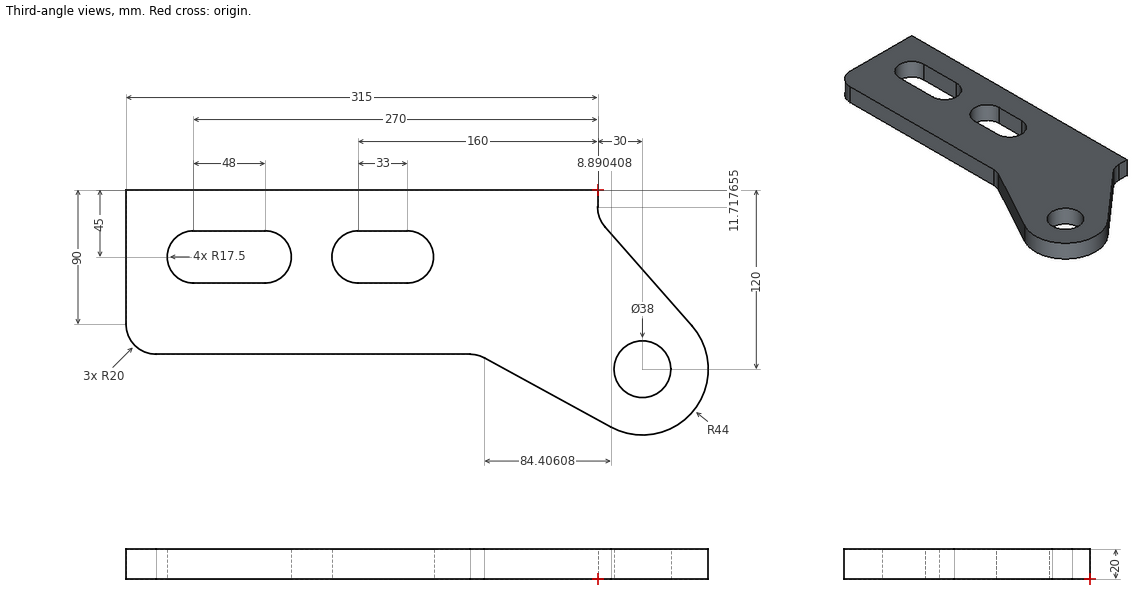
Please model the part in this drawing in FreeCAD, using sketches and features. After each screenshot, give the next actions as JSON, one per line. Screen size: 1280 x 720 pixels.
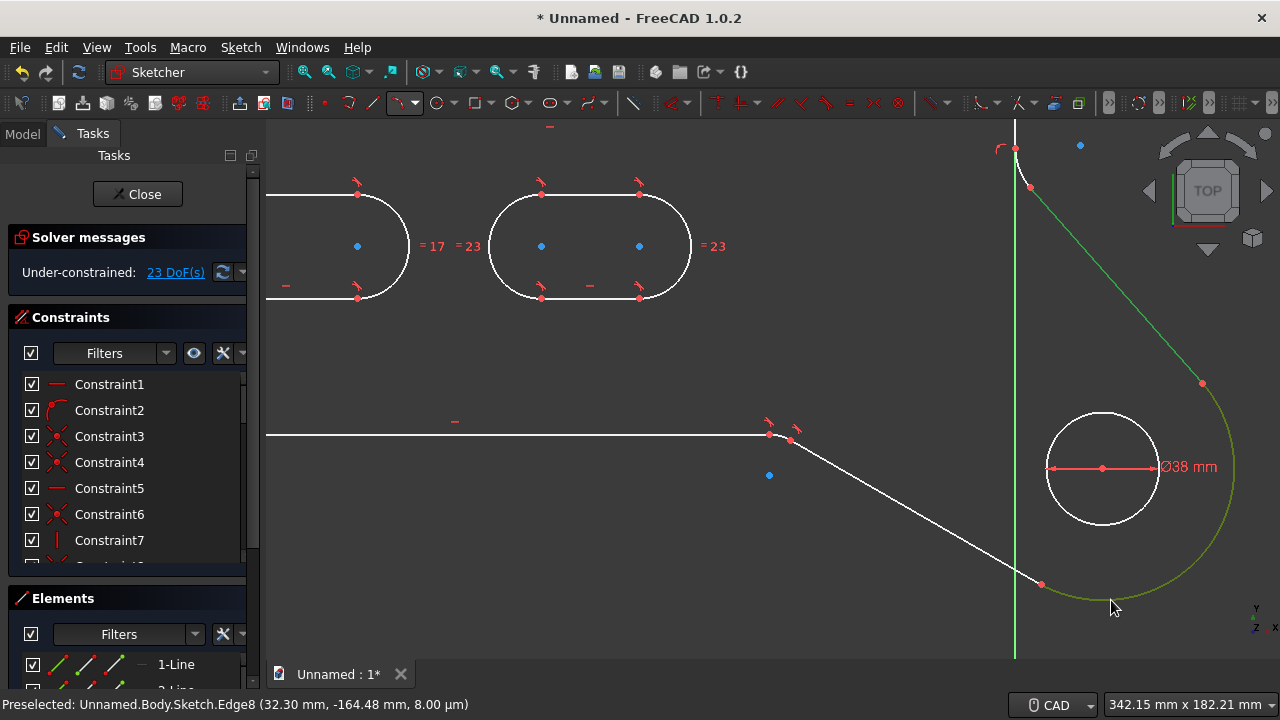
{"action": "left_click", "coordinate": [826, 104]}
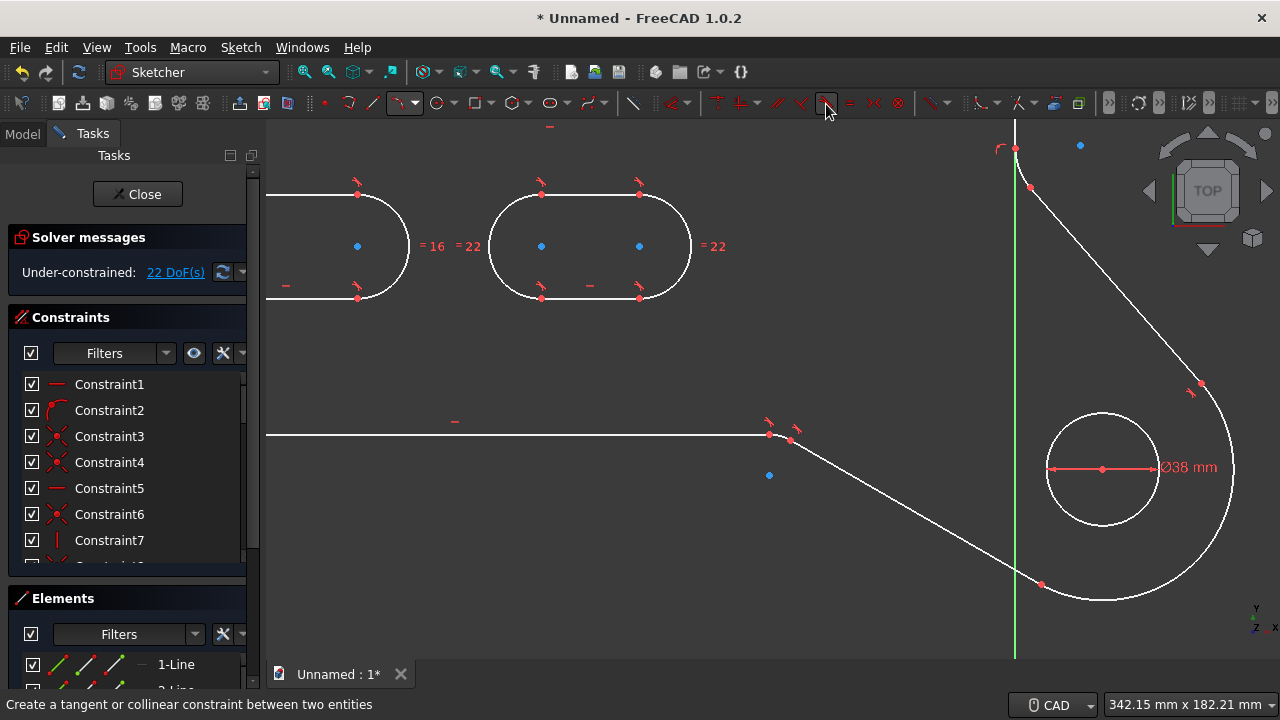
{"action": "left_click", "coordinate": [1081, 246]}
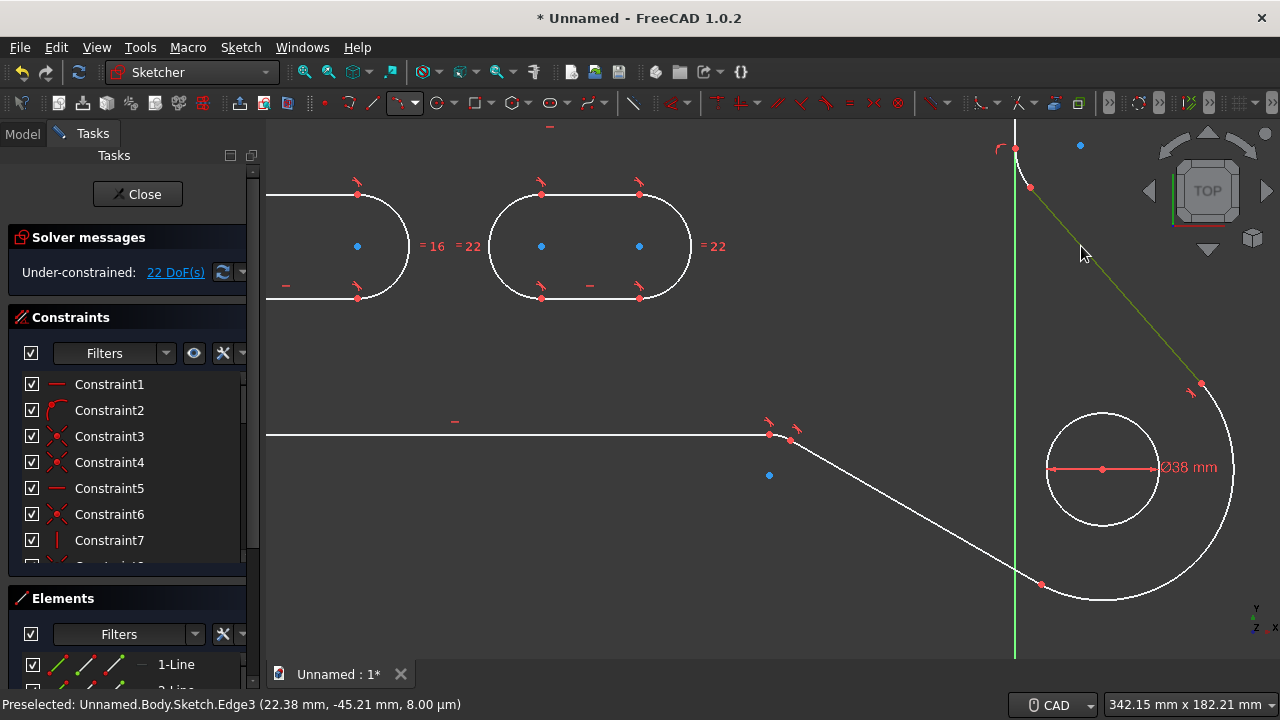
{"action": "left_click", "coordinate": [1017, 161]}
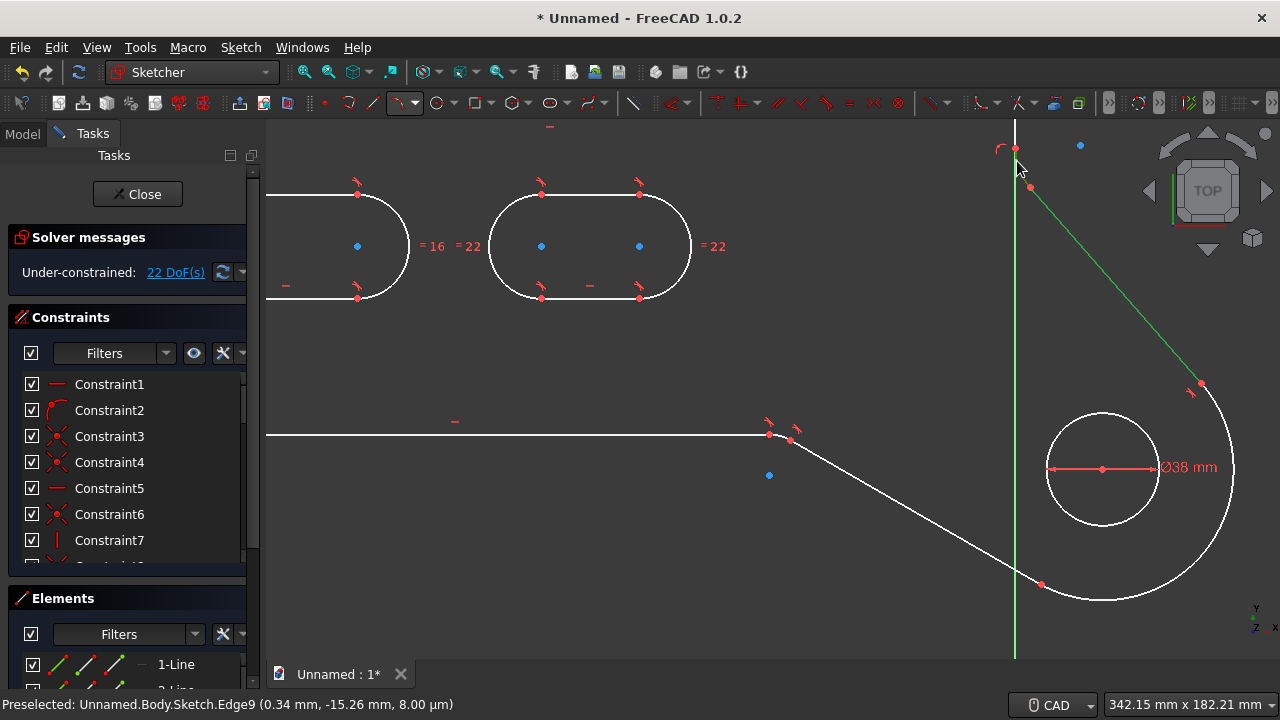
{"action": "key", "text": "t"}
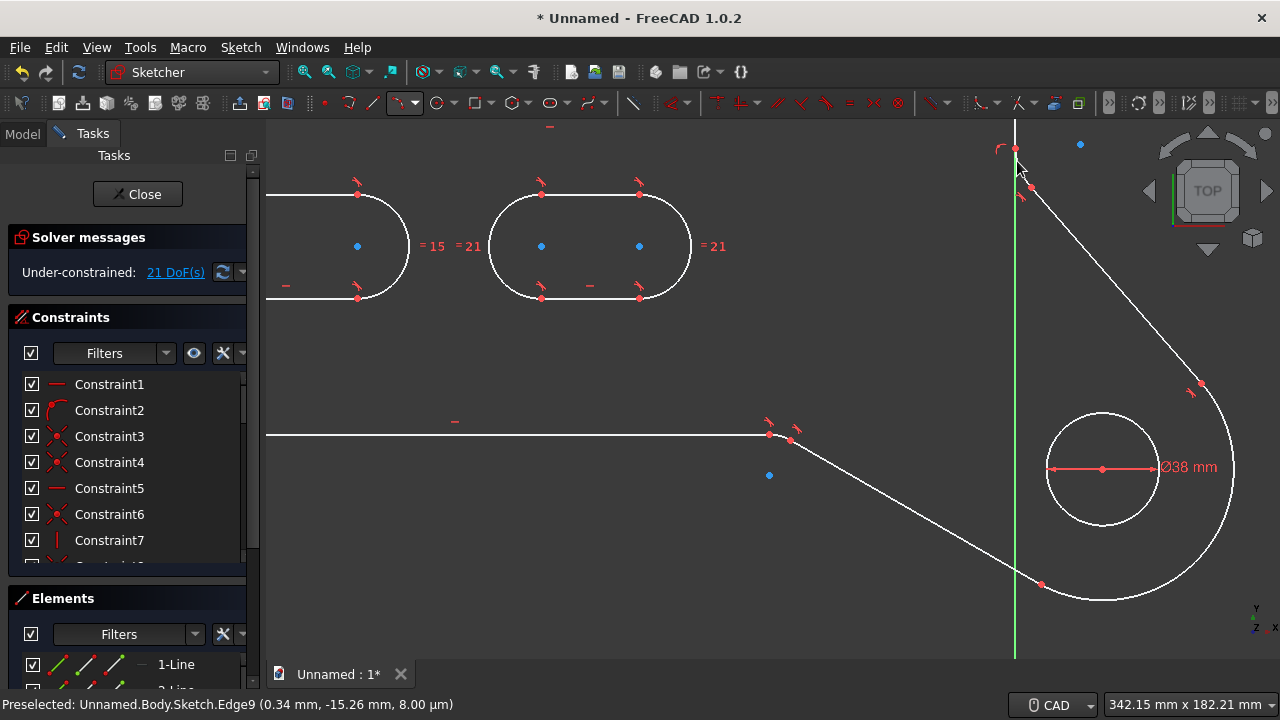
{"action": "scroll", "coordinate": [778, 439], "scroll_direction": "down", "scroll_amount": 3}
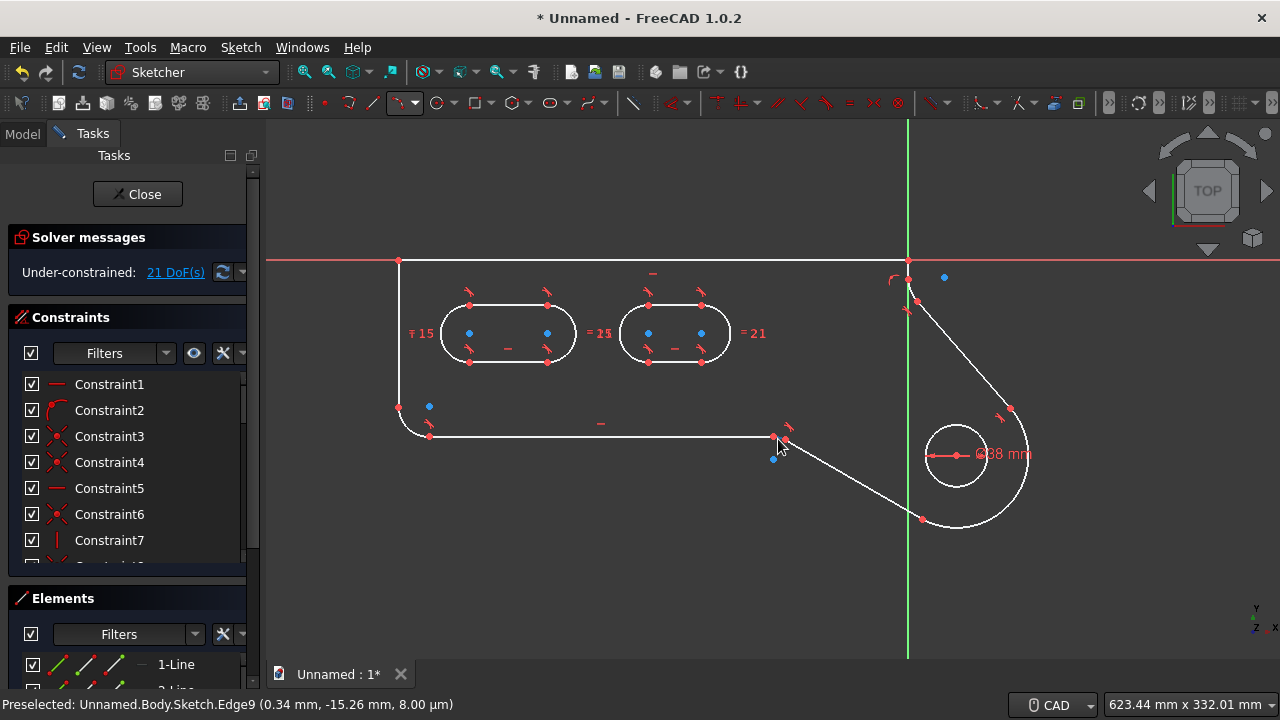
{"action": "scroll", "coordinate": [908, 274], "scroll_direction": "up", "scroll_amount": 5}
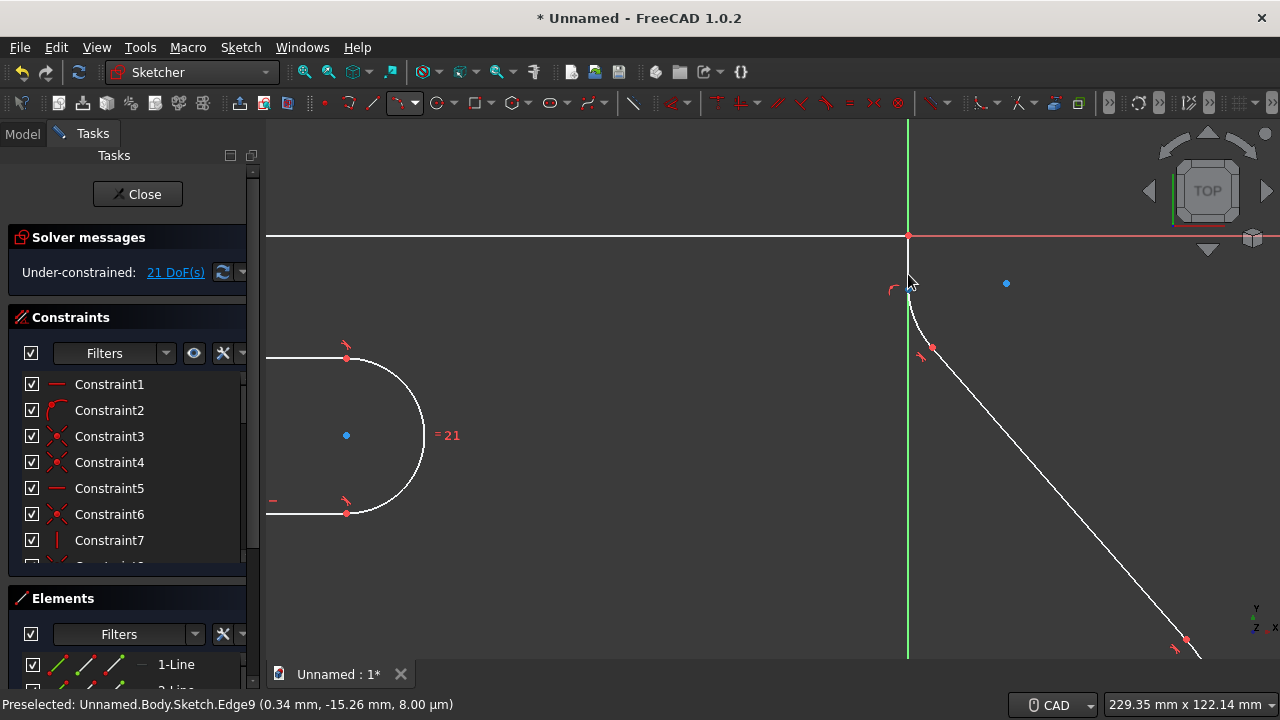
{"action": "left_click", "coordinate": [908, 273]}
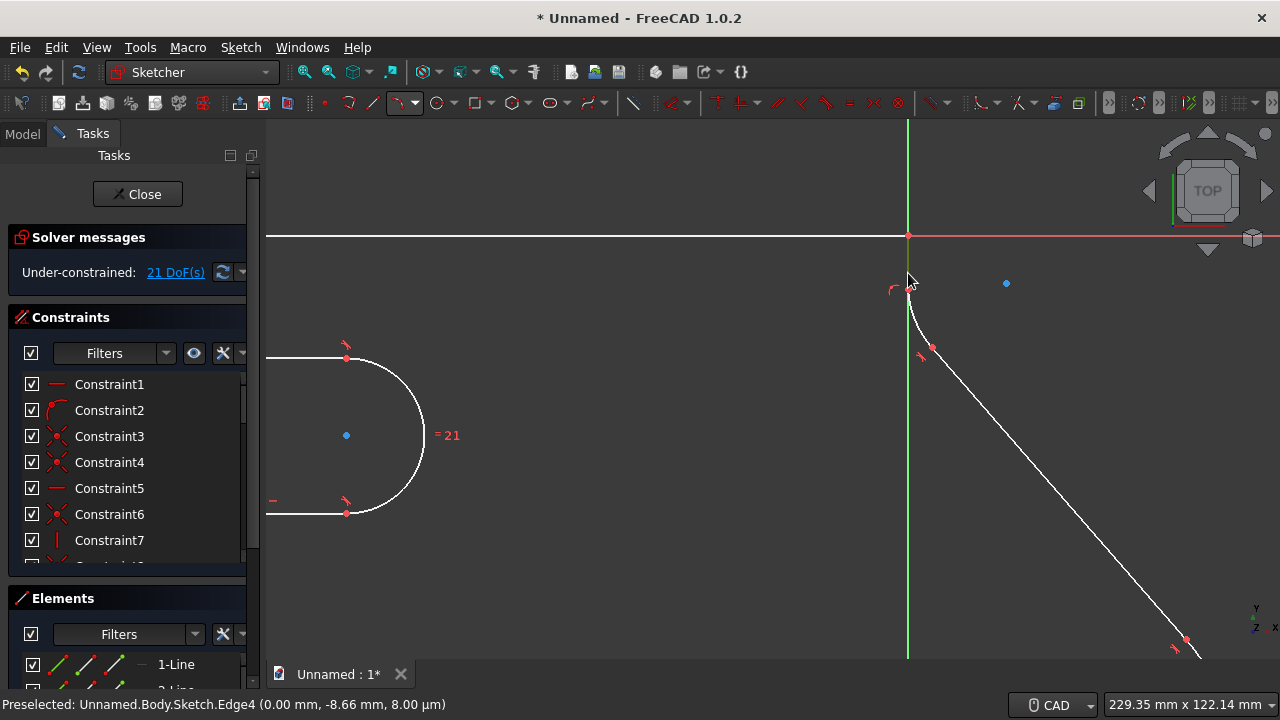
{"action": "left_click", "coordinate": [911, 308]}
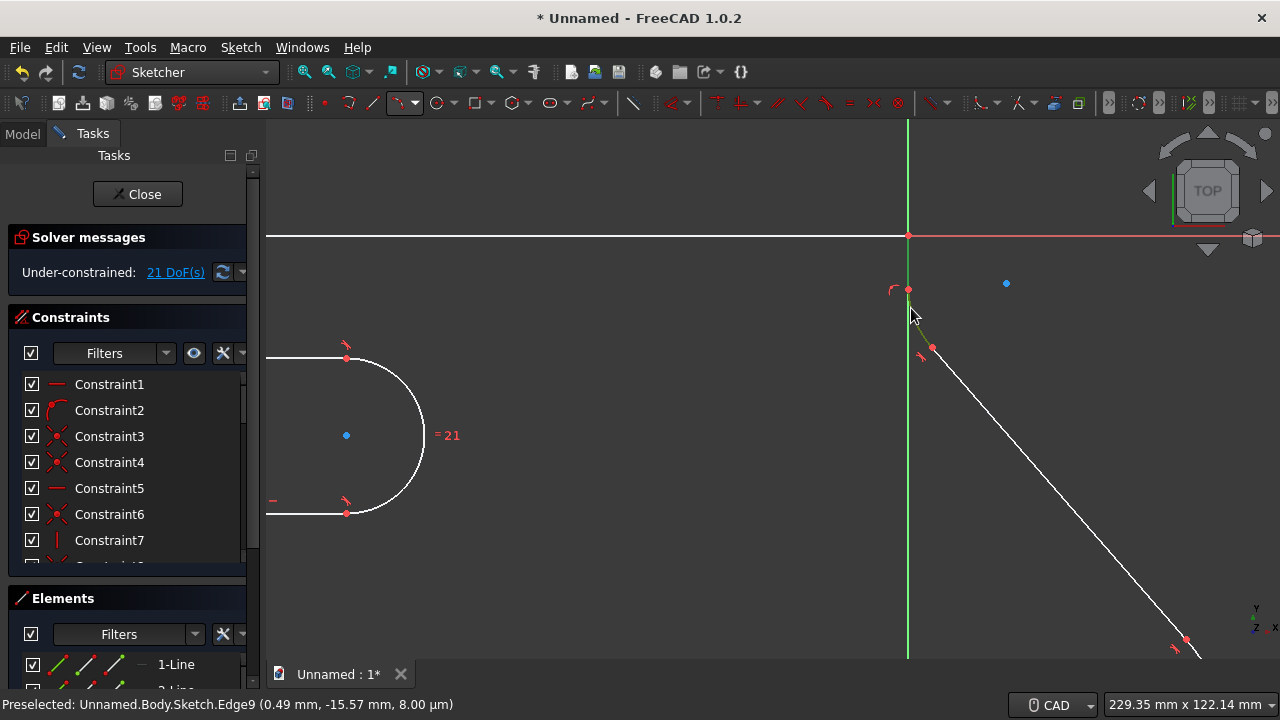
{"action": "key", "text": "t"}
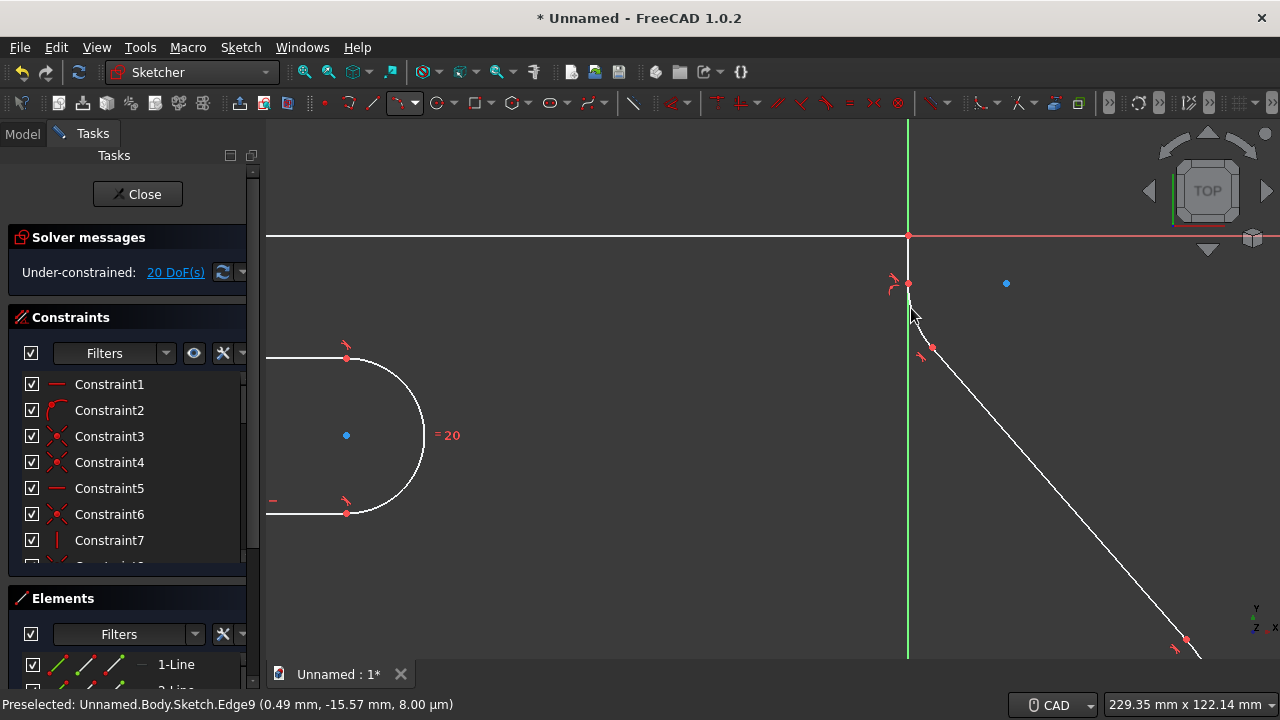
{"action": "scroll", "coordinate": [908, 274], "scroll_direction": "down", "scroll_amount": 5}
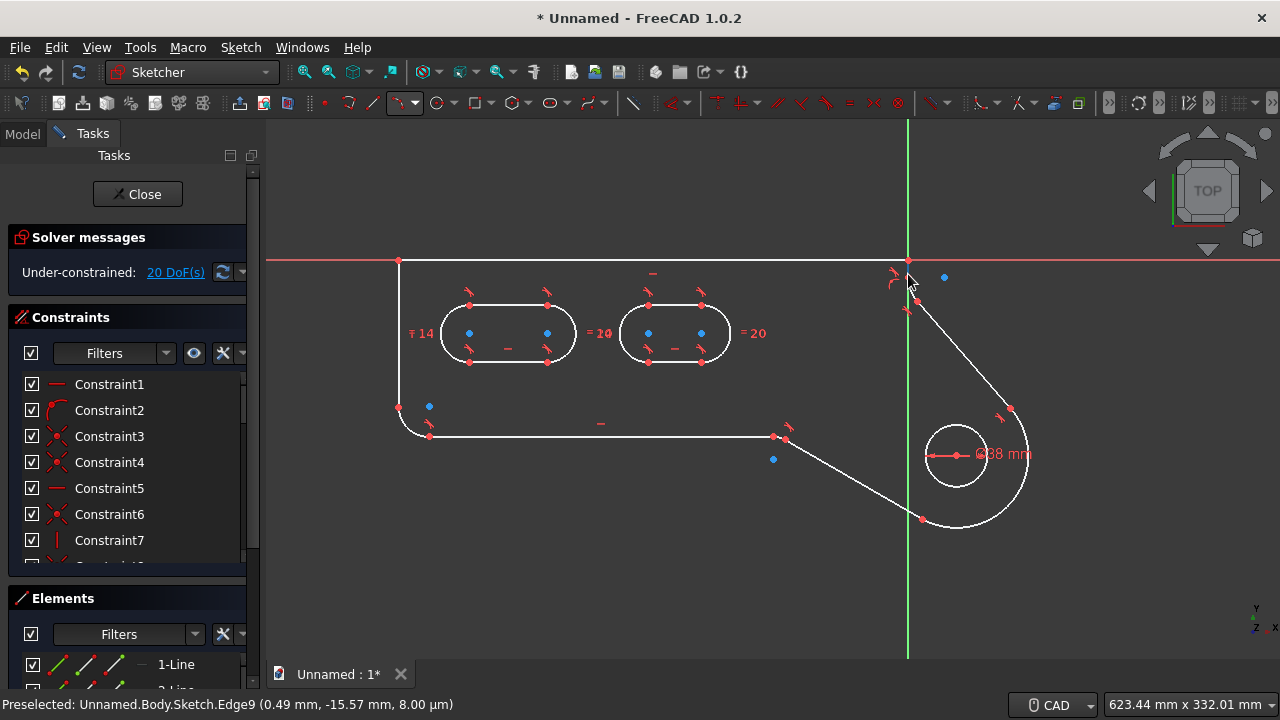
{"action": "left_click", "coordinate": [399, 304]}